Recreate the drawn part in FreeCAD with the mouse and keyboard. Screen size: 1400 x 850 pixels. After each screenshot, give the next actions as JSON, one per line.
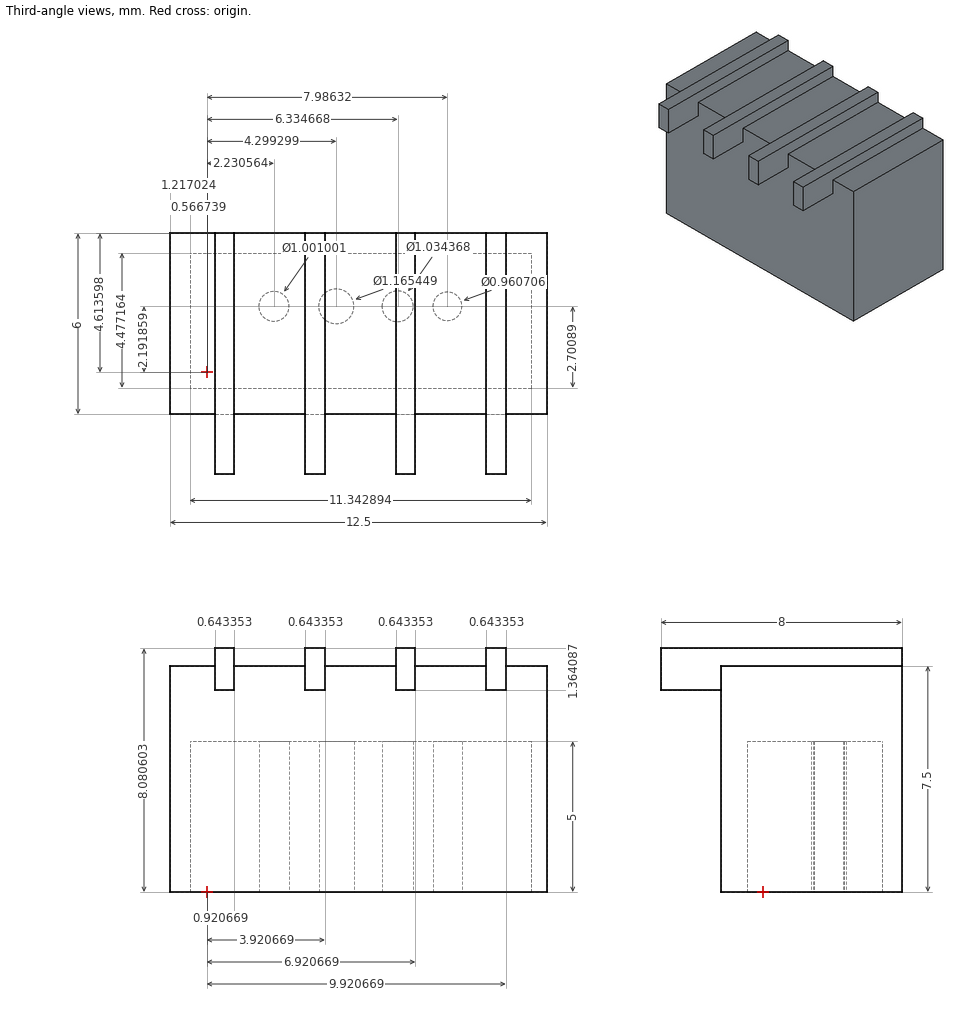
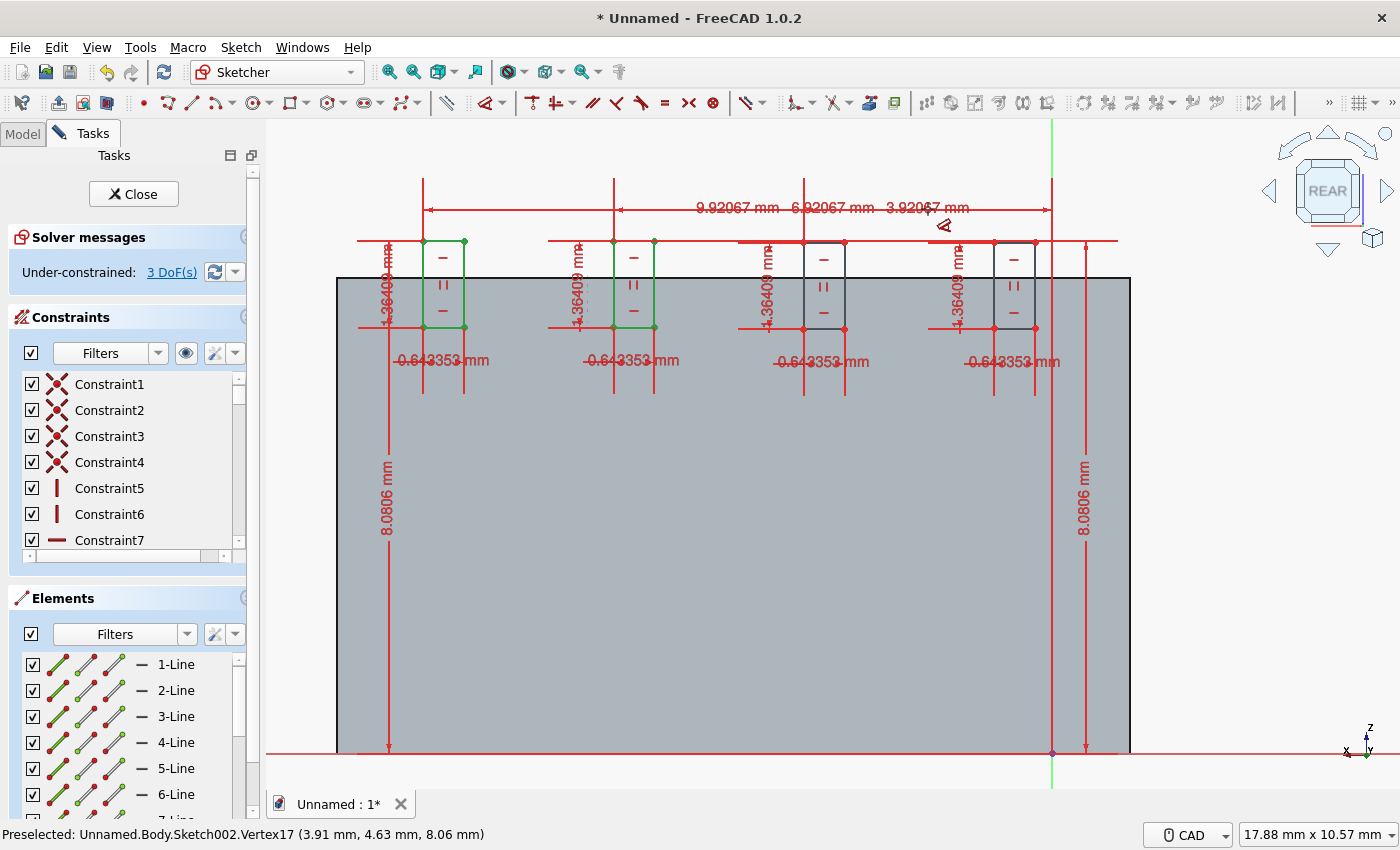
{"action": "left_click", "coordinate": [804, 243]}
{"action": "left_click", "coordinate": [1086, 381]}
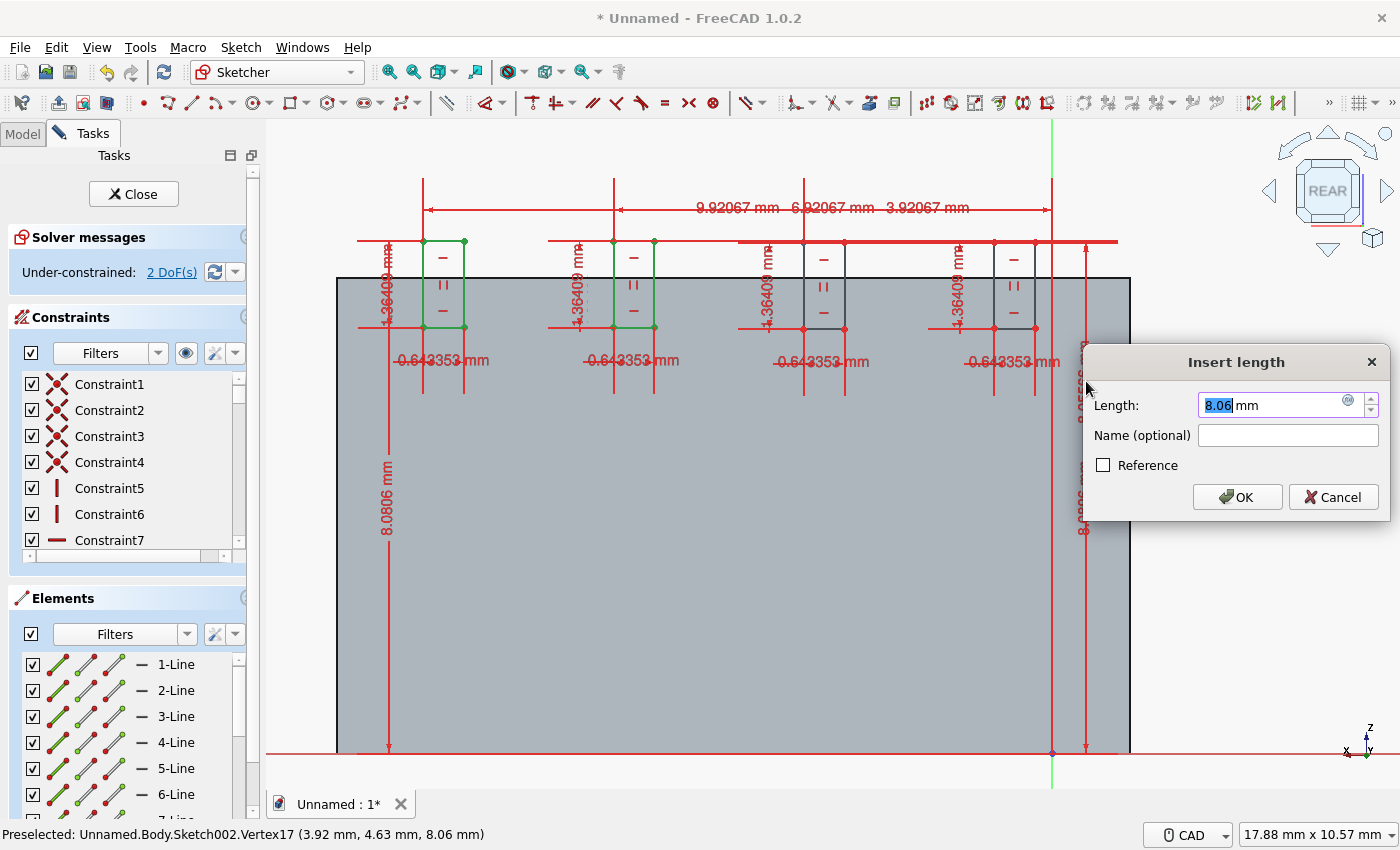
{"action": "type", "text": "8.080603"}
{"action": "key", "text": "Return"}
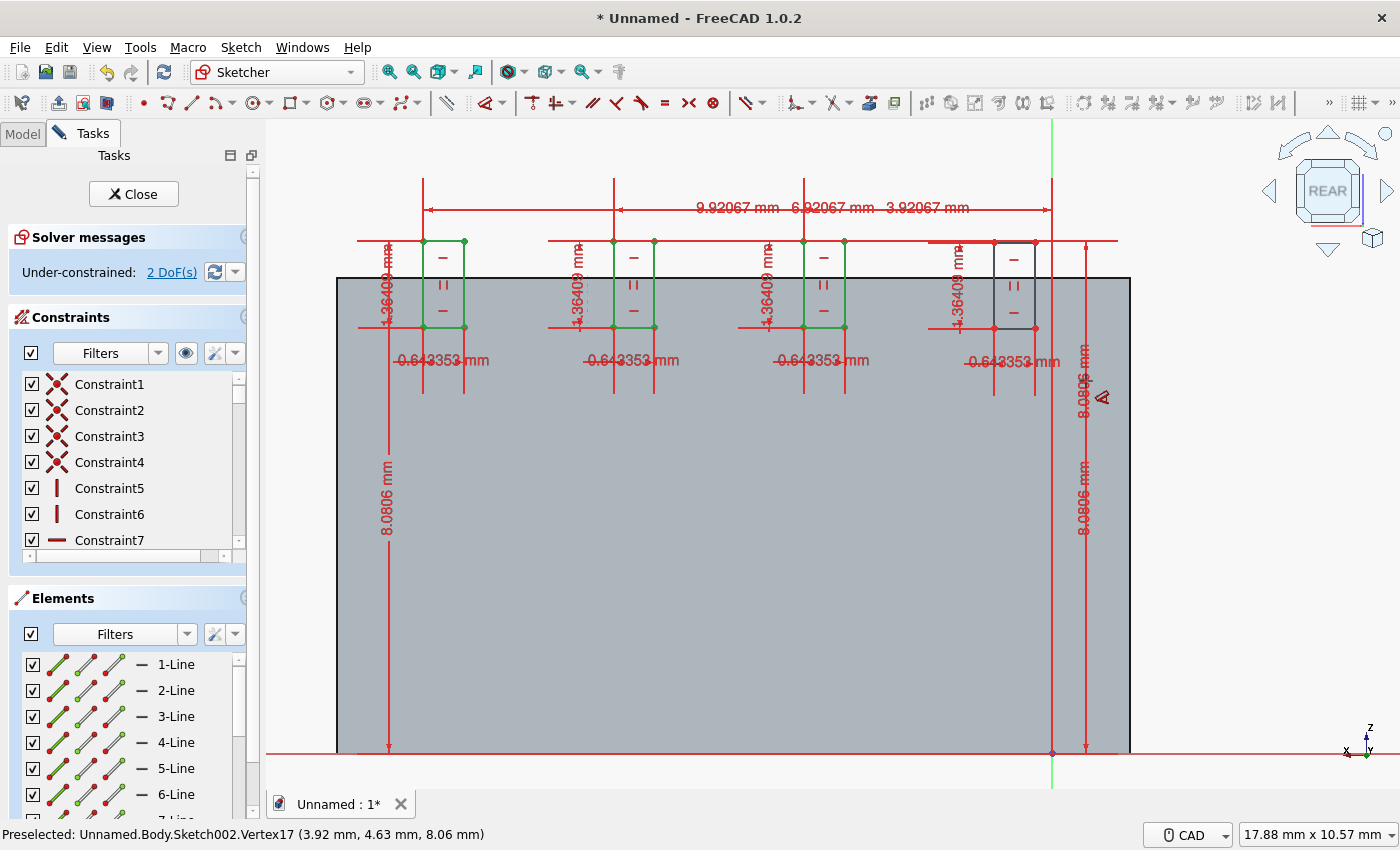
{"action": "left_click", "coordinate": [994, 243]}
{"action": "left_click", "coordinate": [1023, 209]}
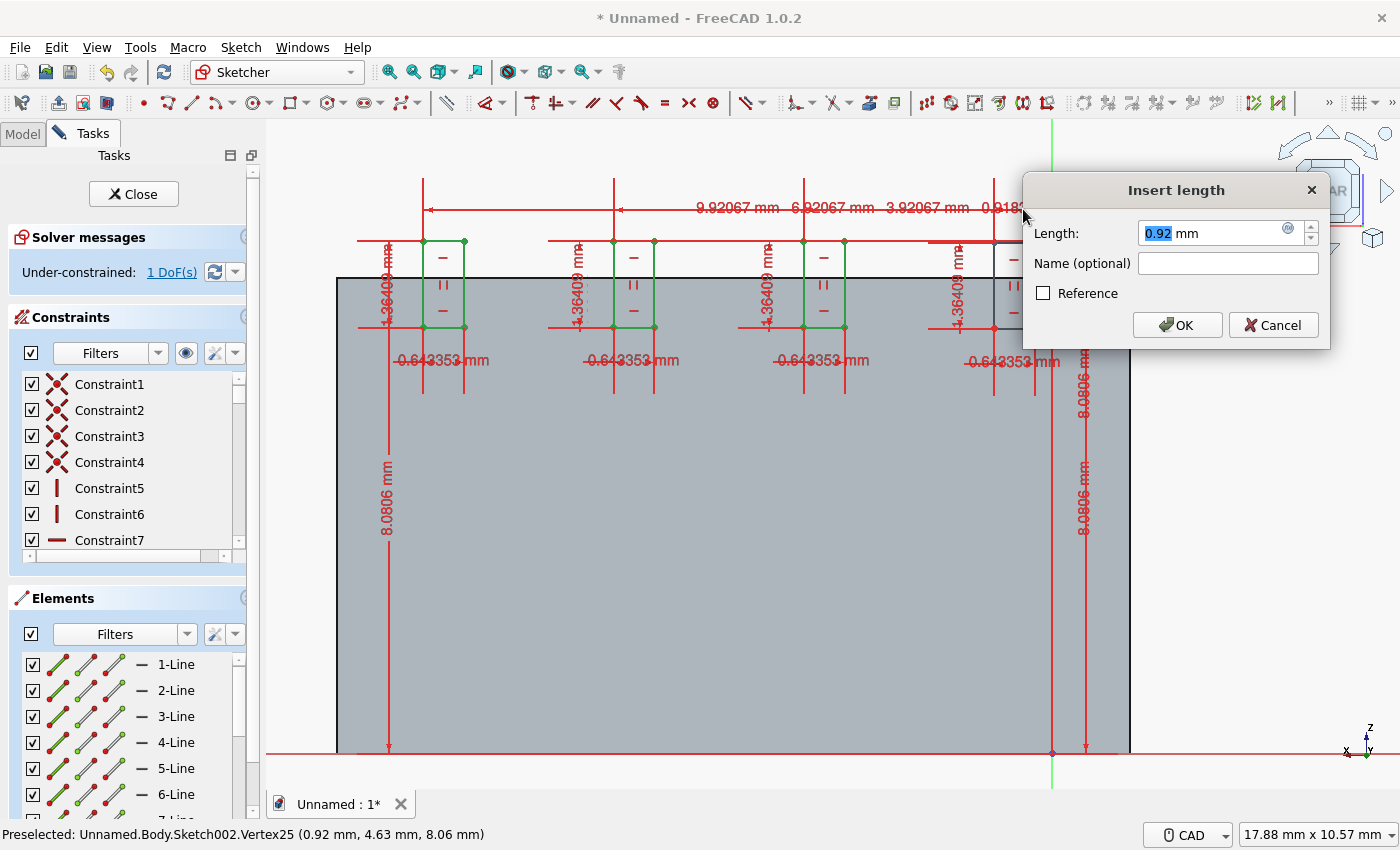
{"action": "type", "text": "0.920669"}
{"action": "key", "text": "Return"}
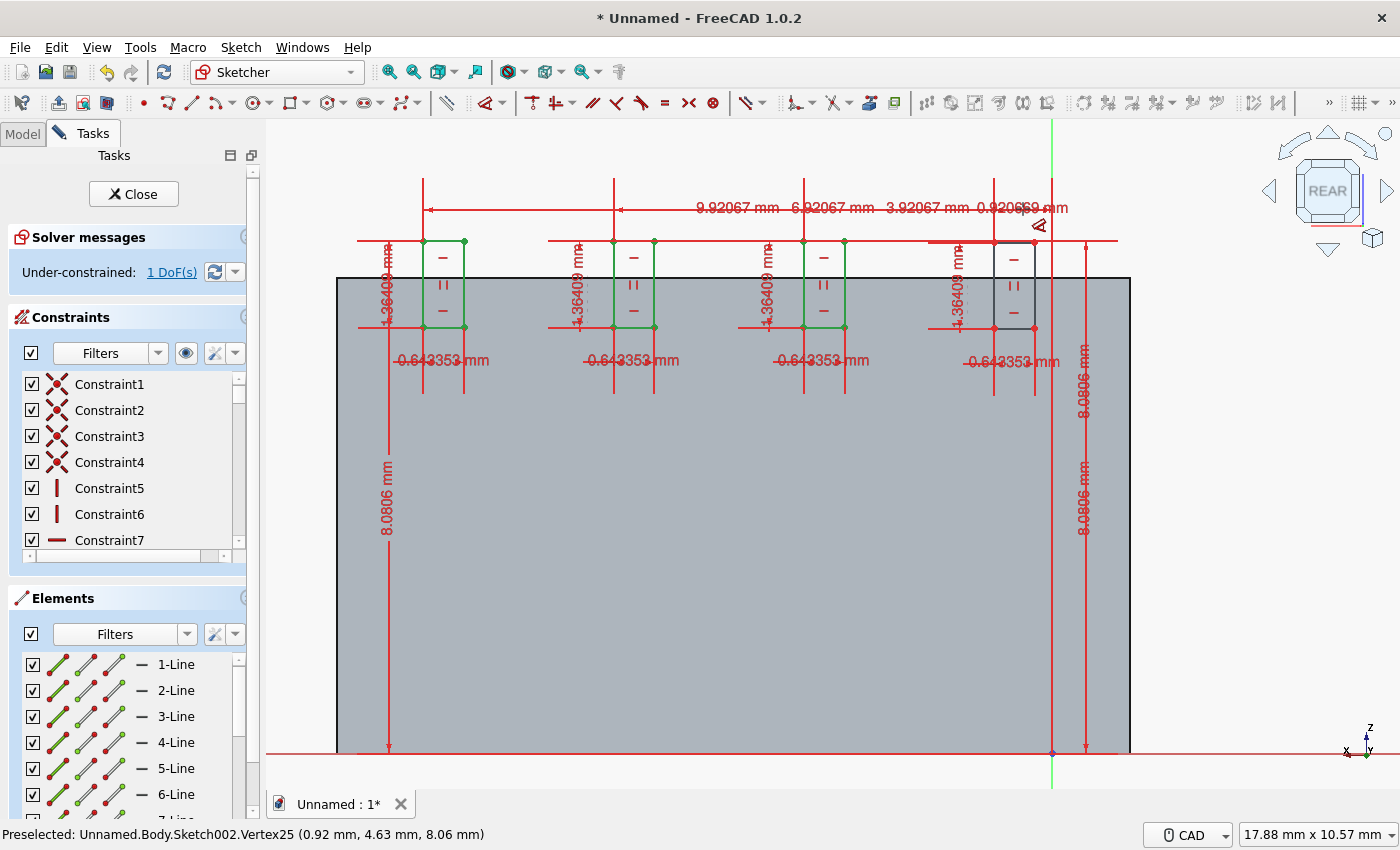
{"action": "left_click", "coordinate": [994, 243]}
{"action": "left_click", "coordinate": [1086, 616]}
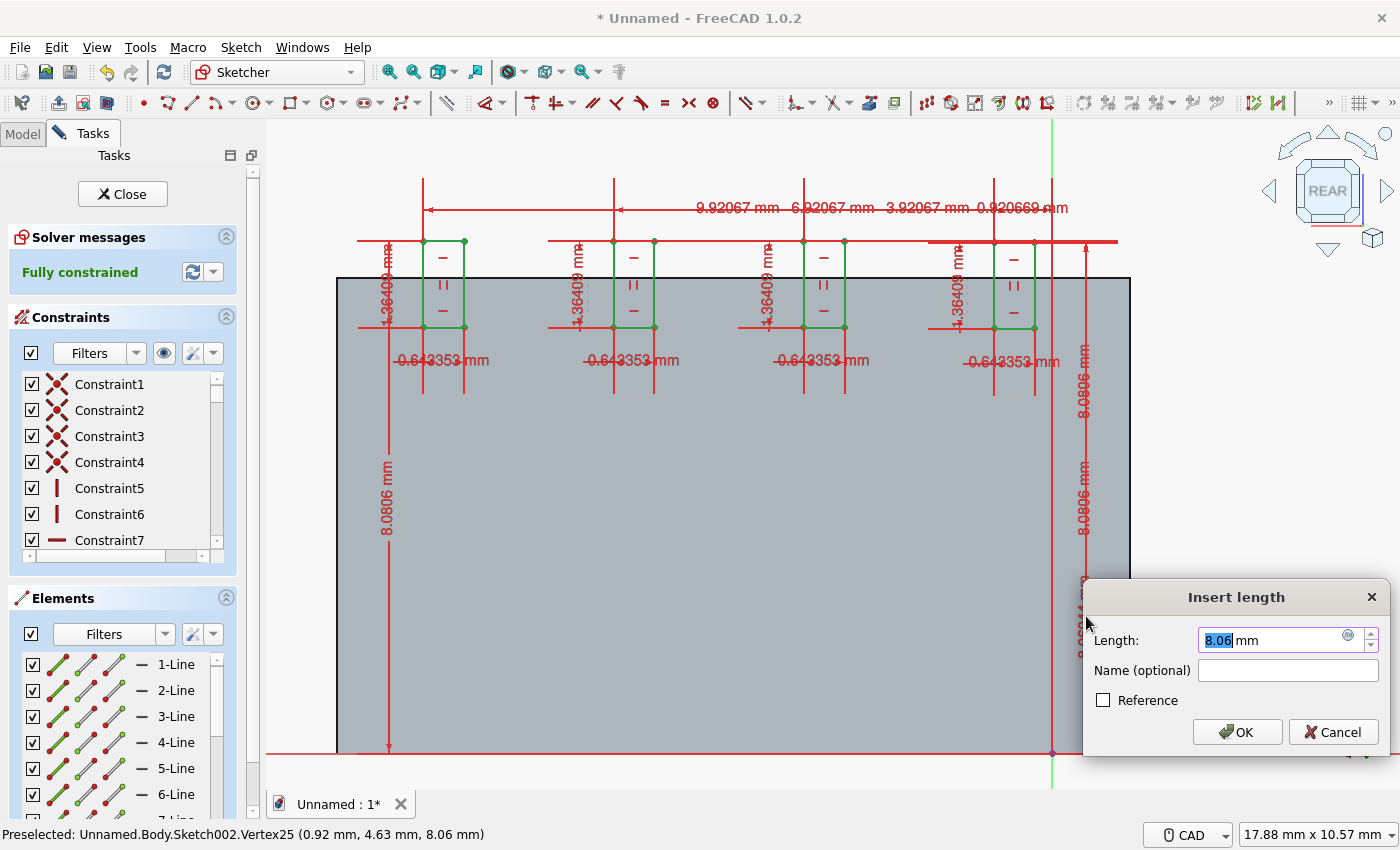
{"action": "type", "text": "8.080603"}
{"action": "key", "text": "Return"}
{"action": "key", "text": "Escape"}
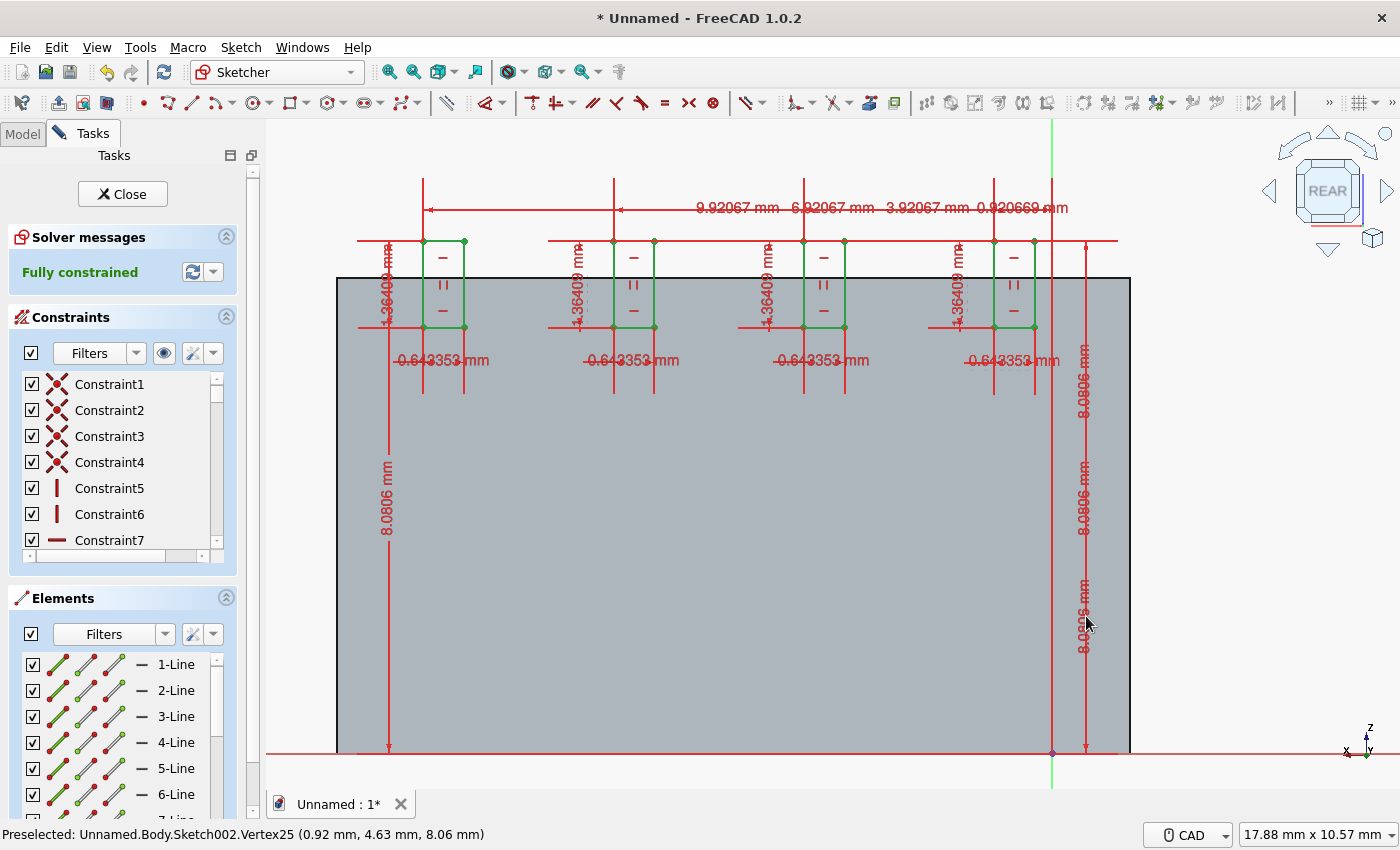
{"action": "left_click", "coordinate": [123, 194]}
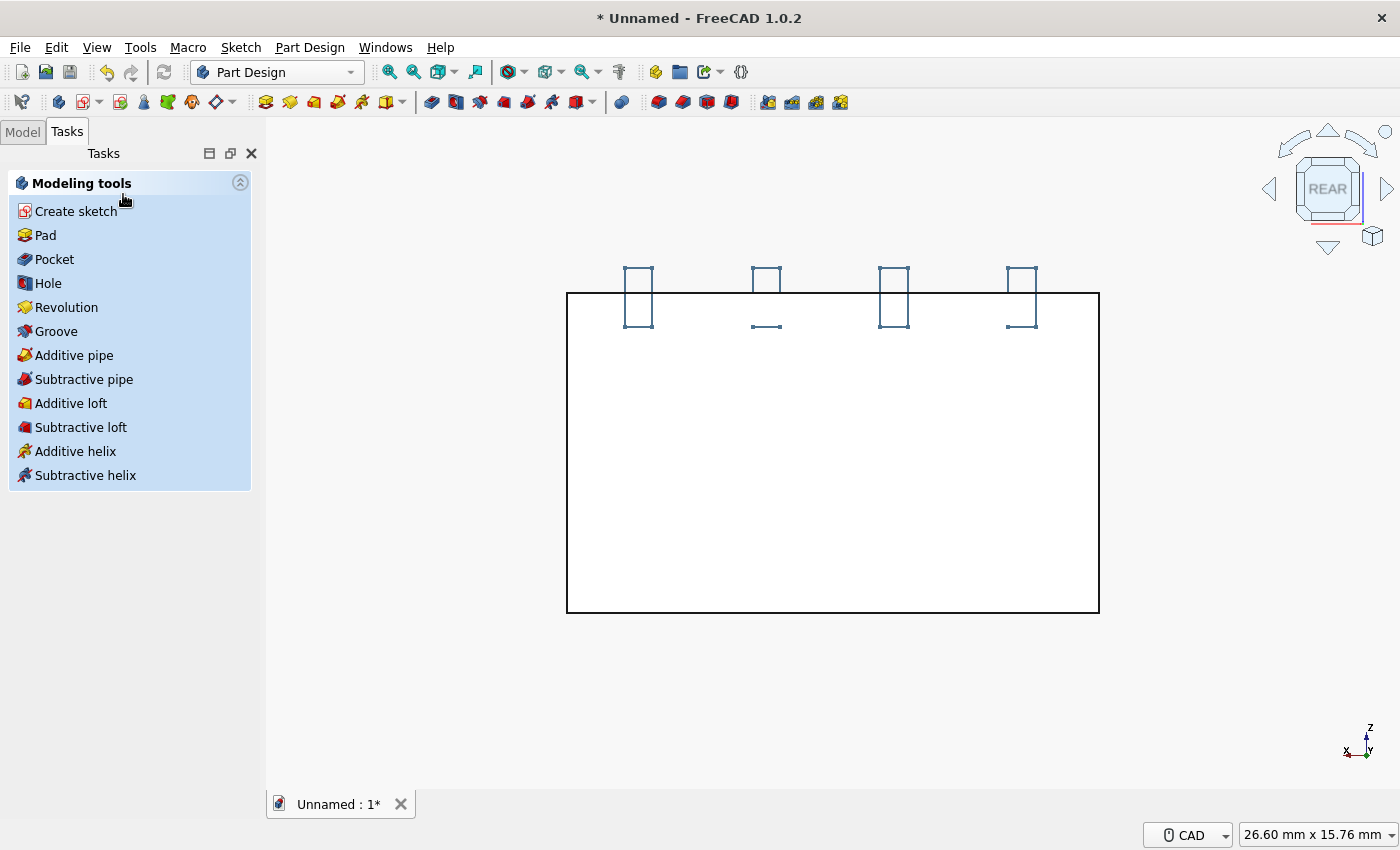
{"action": "left_click", "coordinate": [266, 102]}